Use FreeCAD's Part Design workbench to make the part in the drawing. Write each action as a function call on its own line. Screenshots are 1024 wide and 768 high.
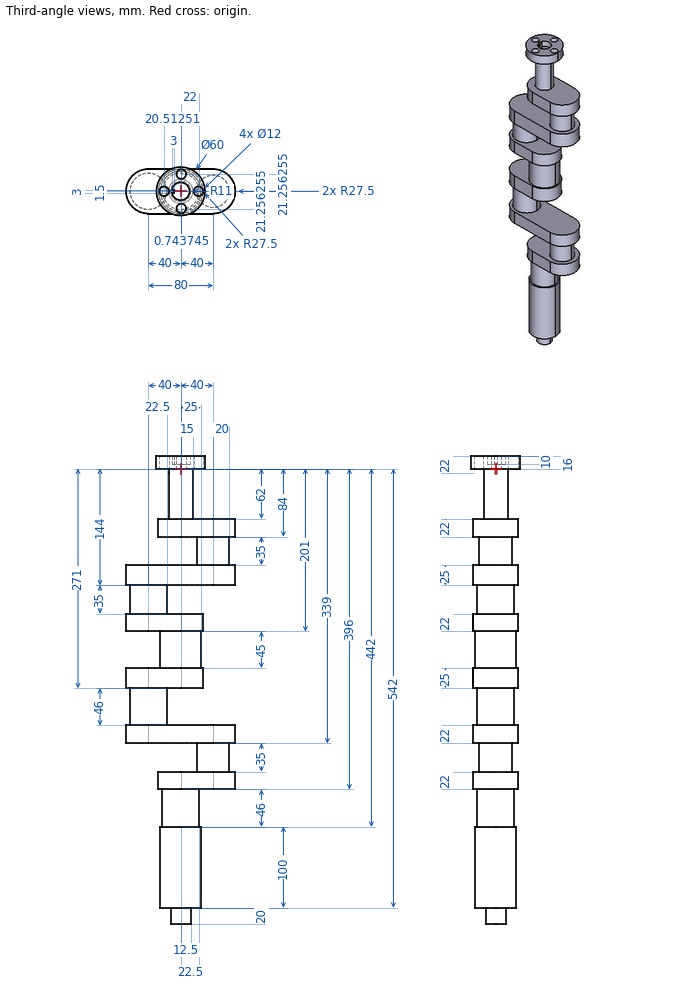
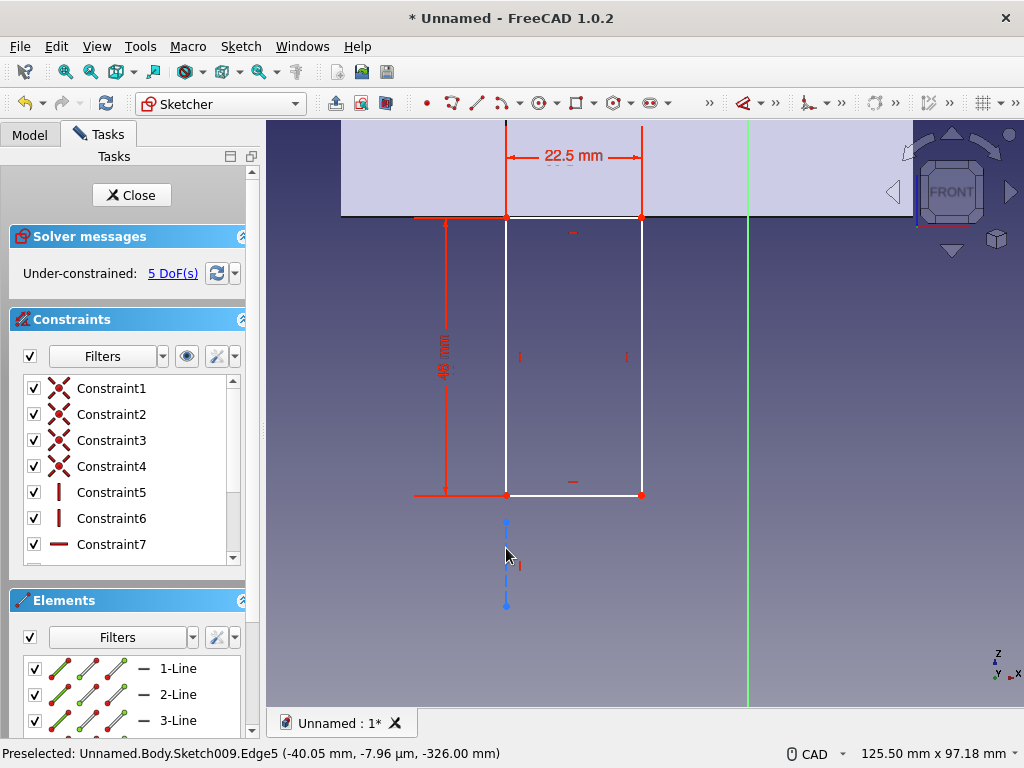
key(d)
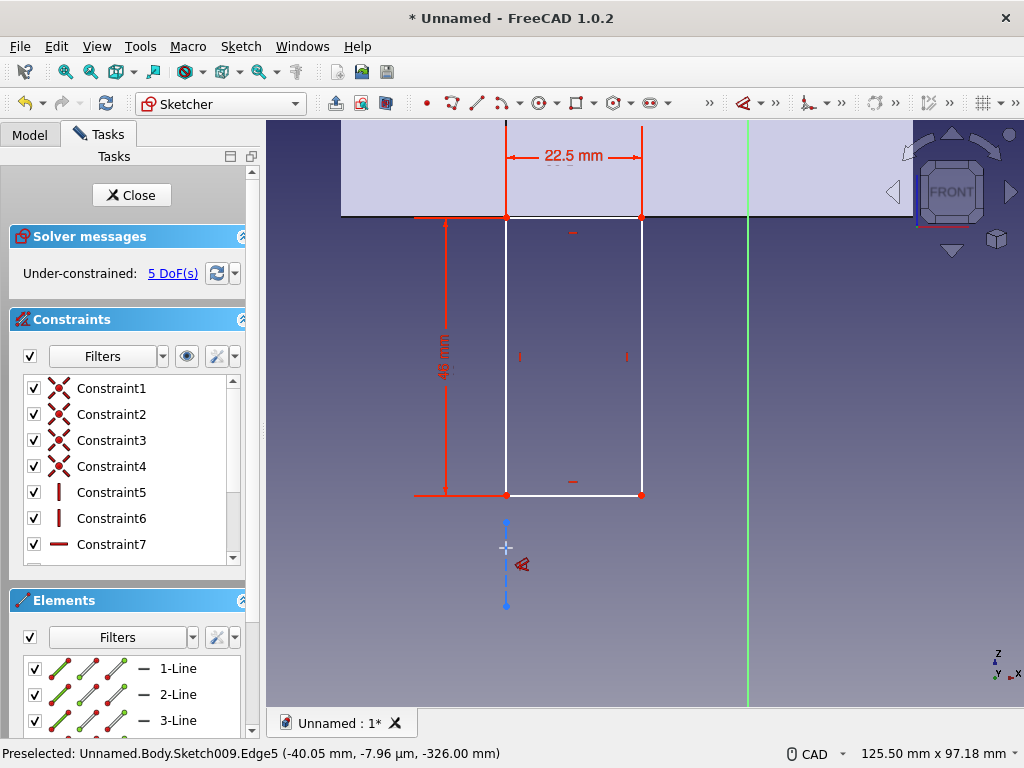
click(506, 218)
click(627, 252)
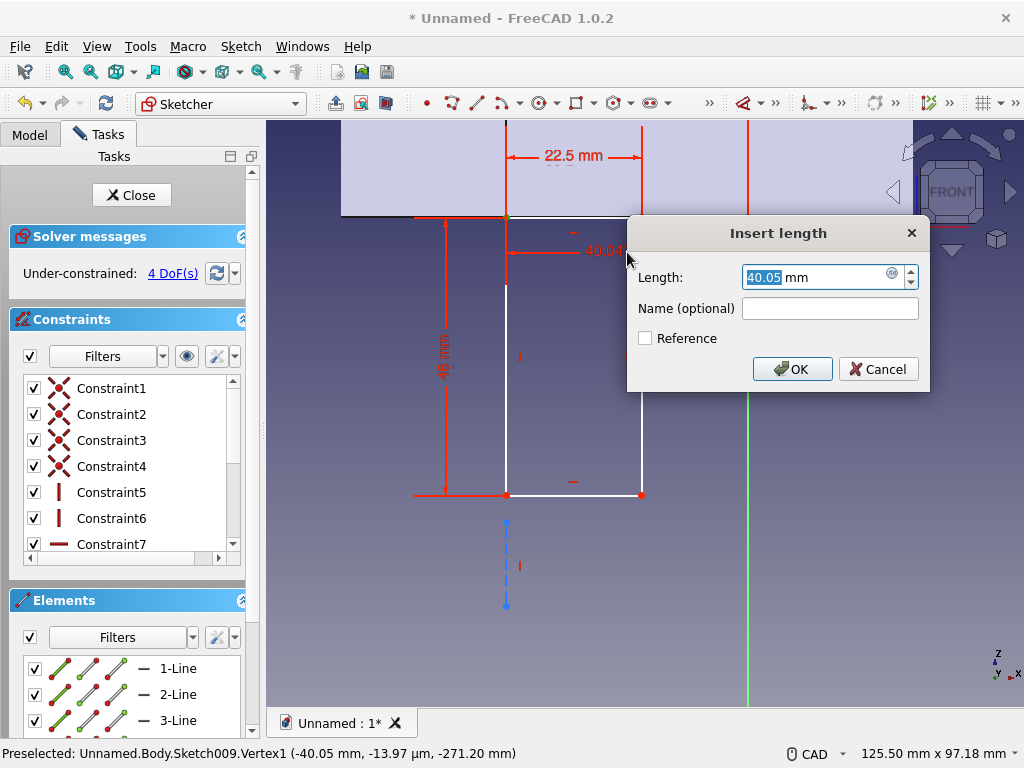
text(40)
key(Return)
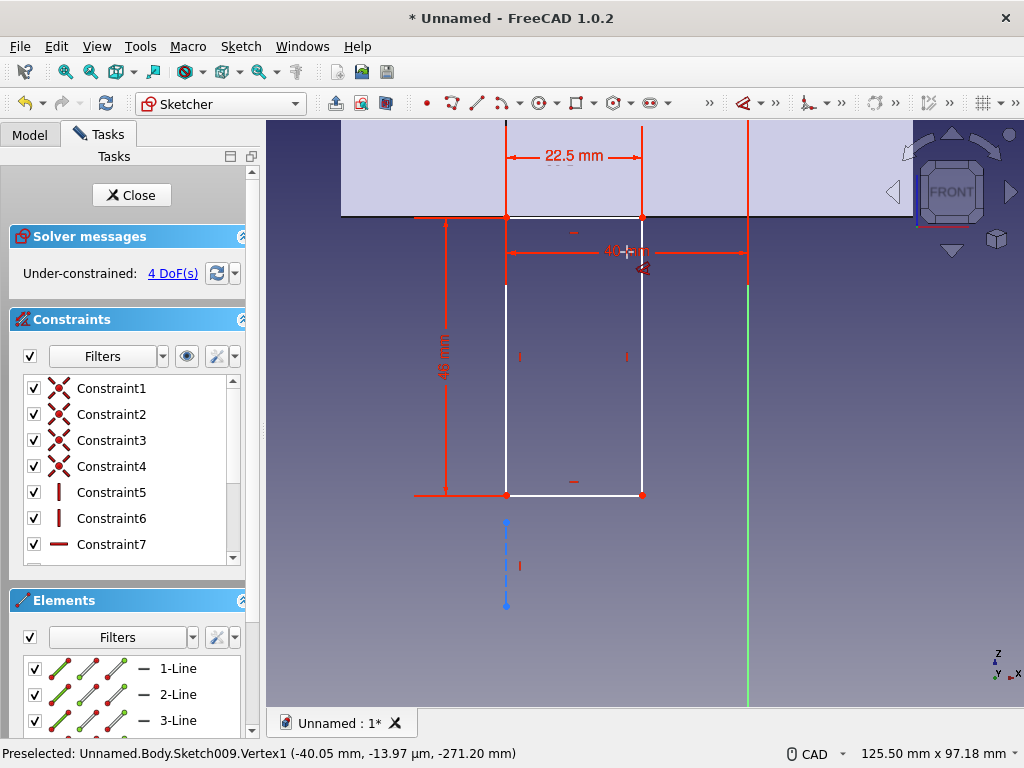
click(506, 523)
click(627, 557)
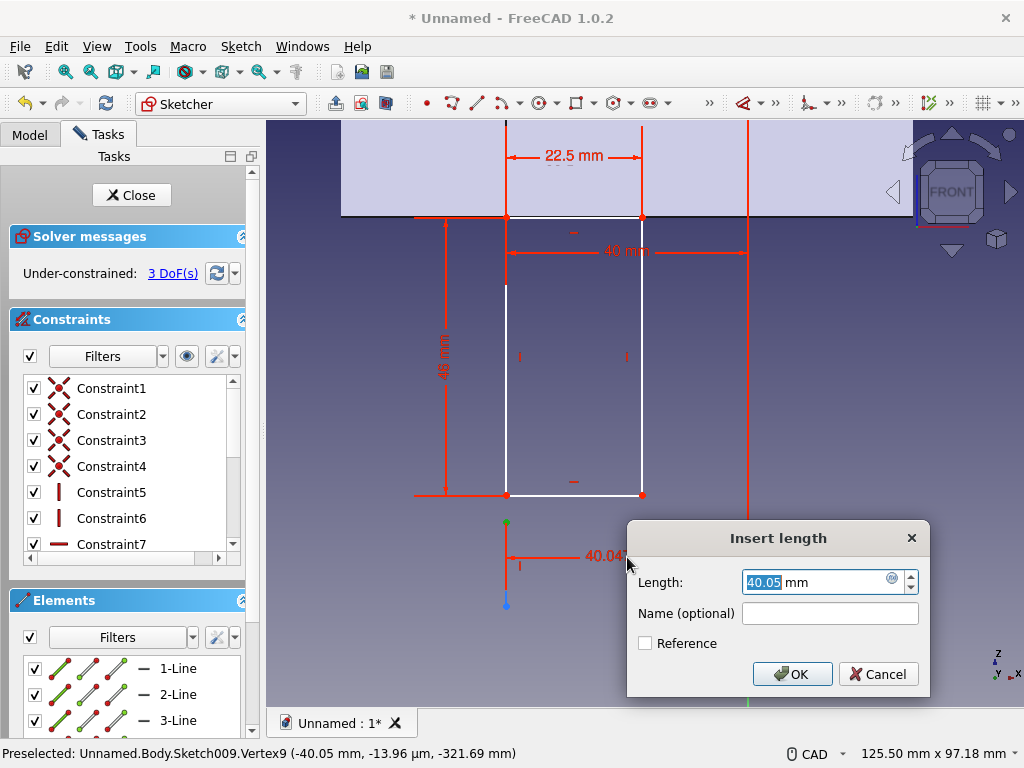
text(40)
key(Return)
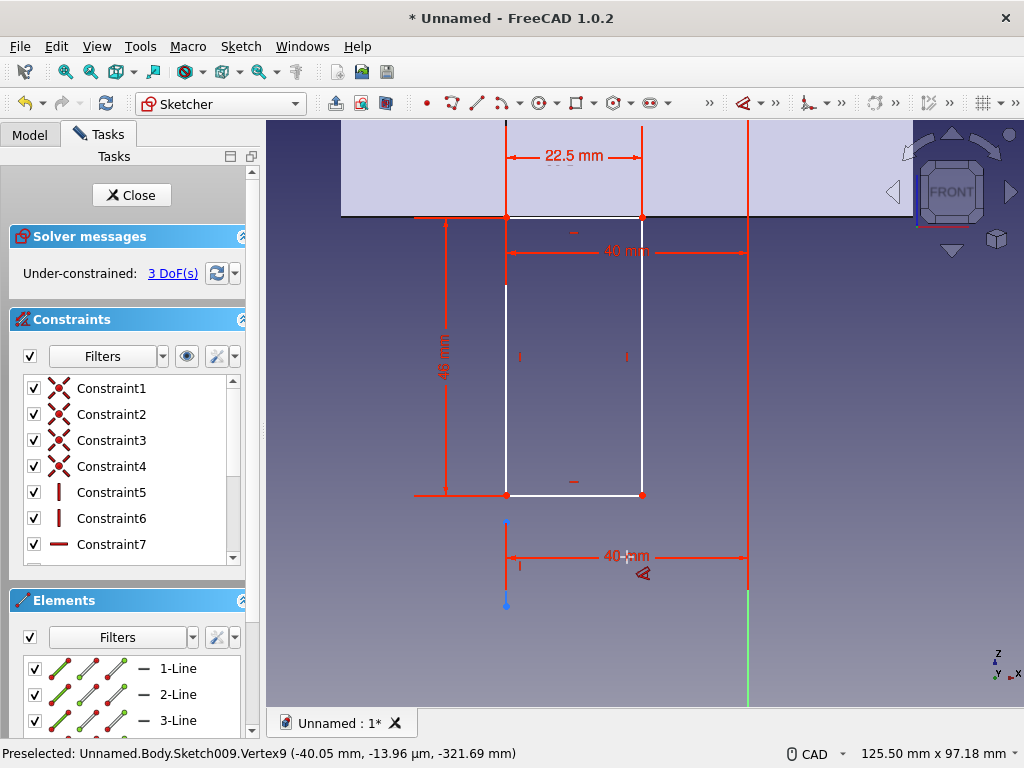
click(506, 218)
click(782, 183)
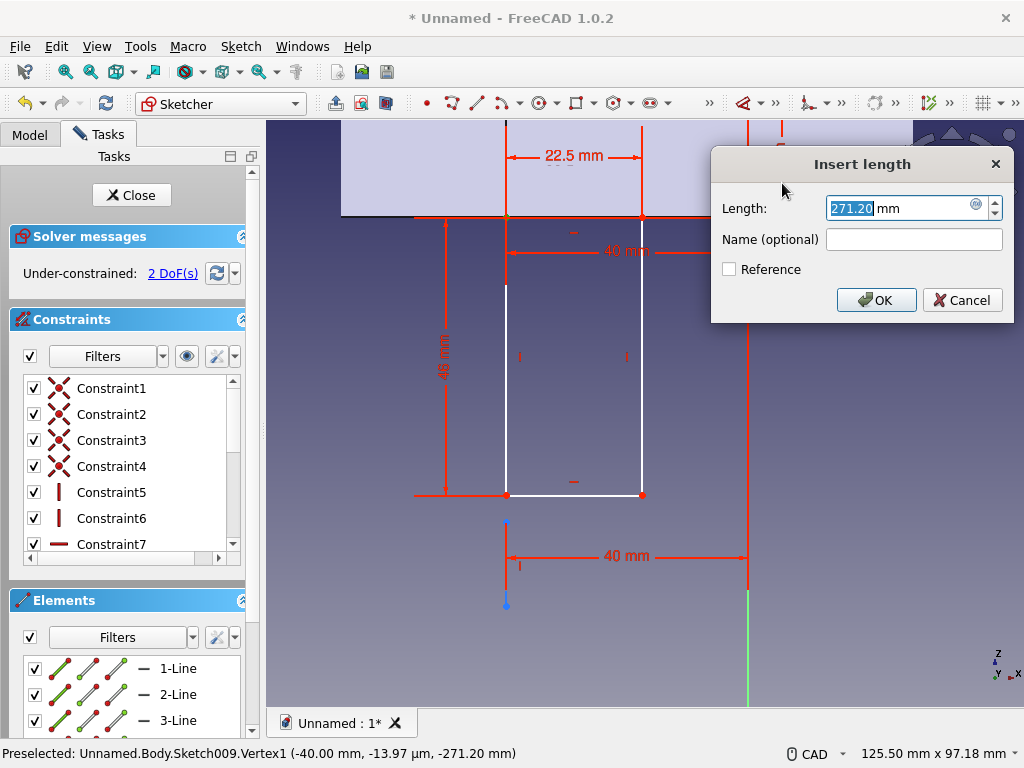
text(271)
key(Return)
key(Escape)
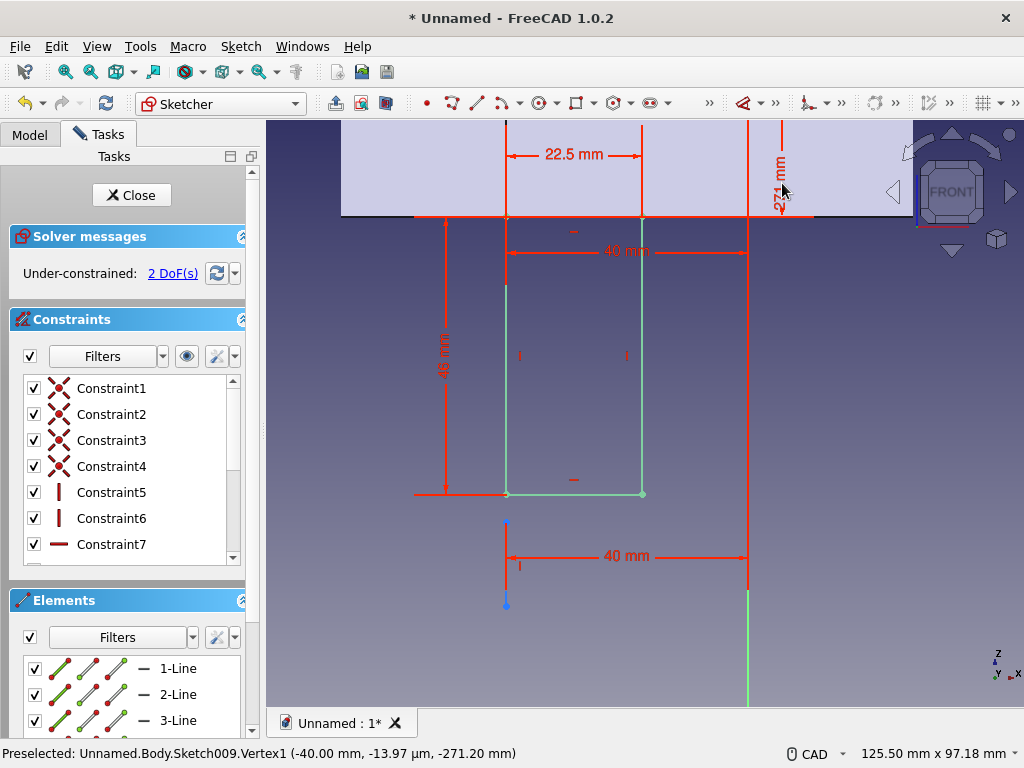
click(132, 195)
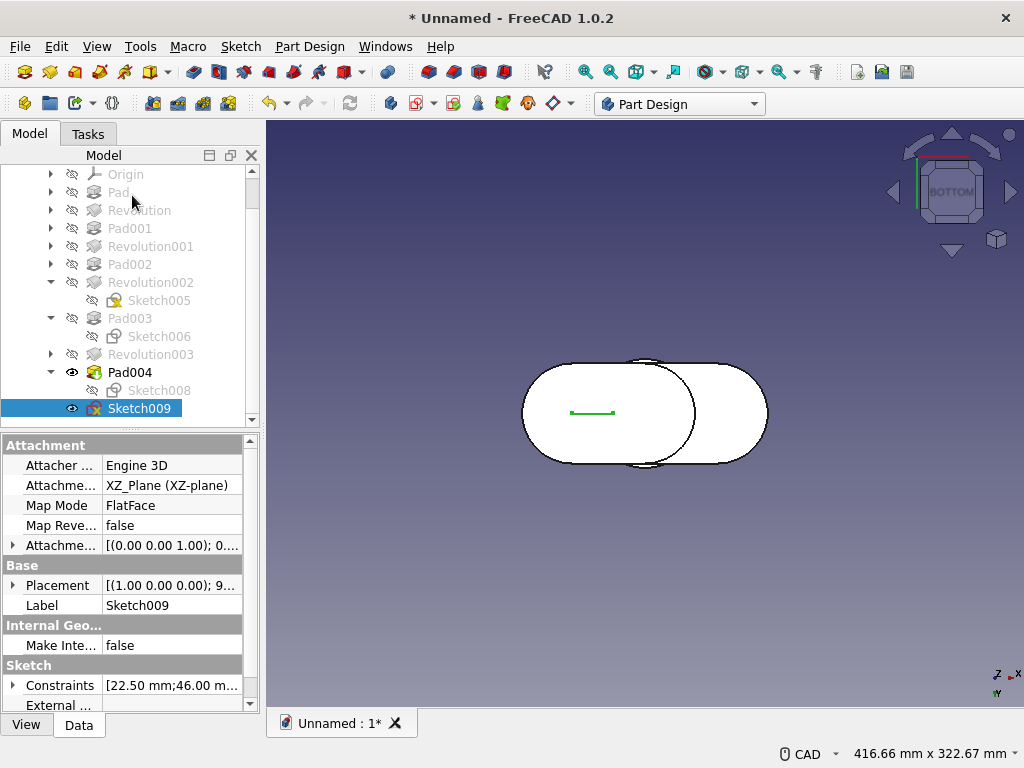
click(50, 72)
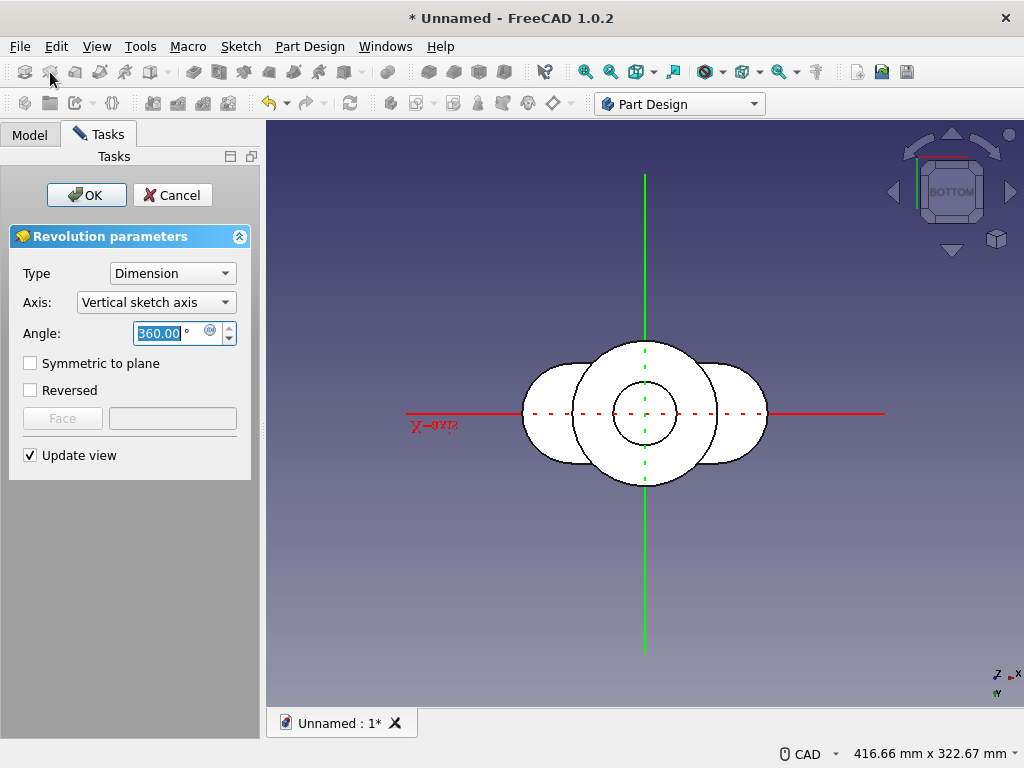
click(157, 302)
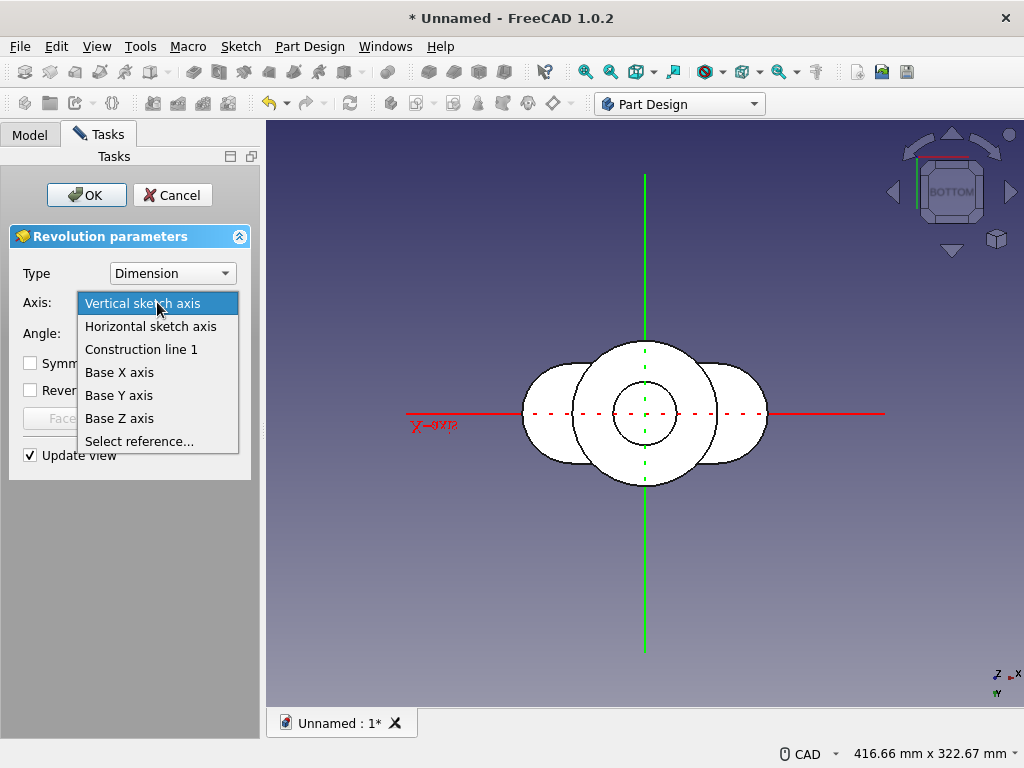
click(156, 350)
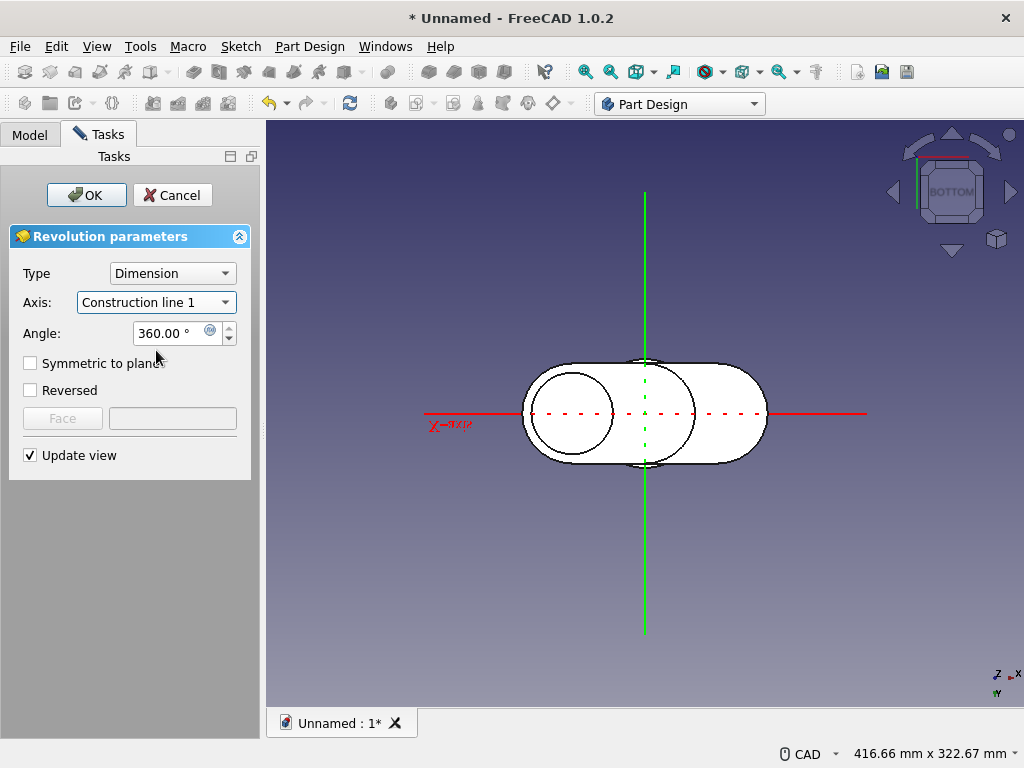
click(87, 195)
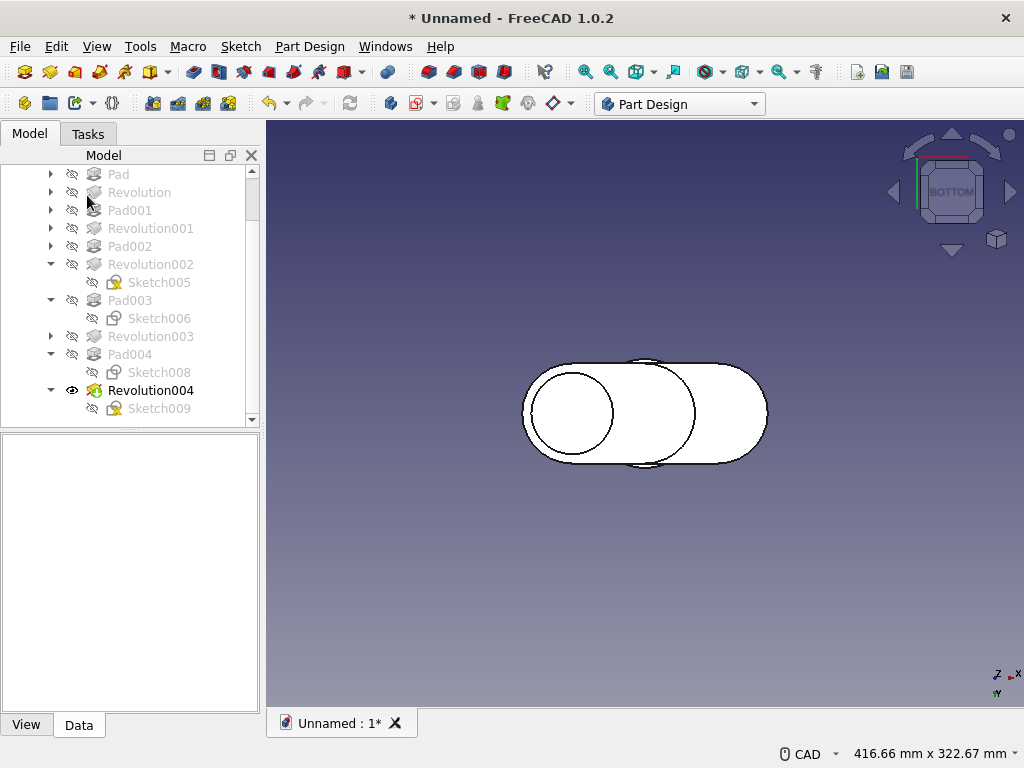
key(v)
key(f)